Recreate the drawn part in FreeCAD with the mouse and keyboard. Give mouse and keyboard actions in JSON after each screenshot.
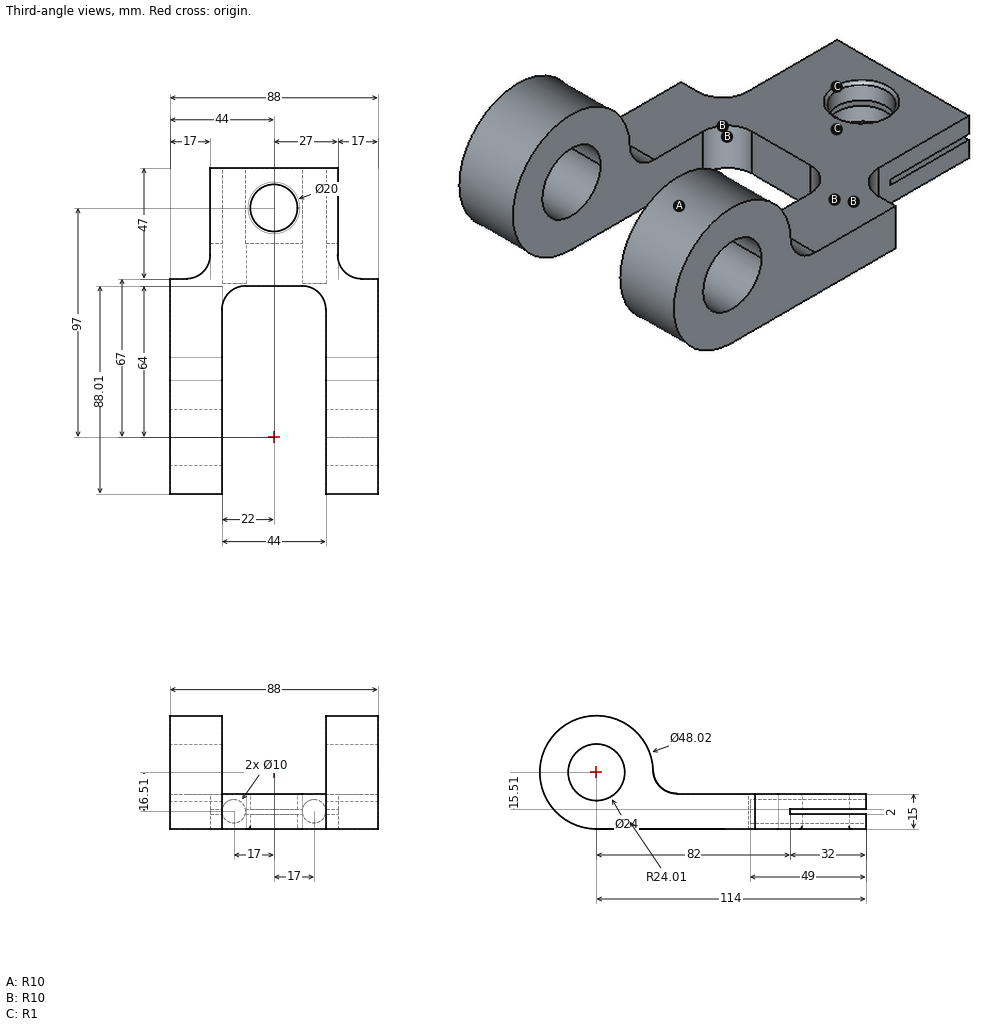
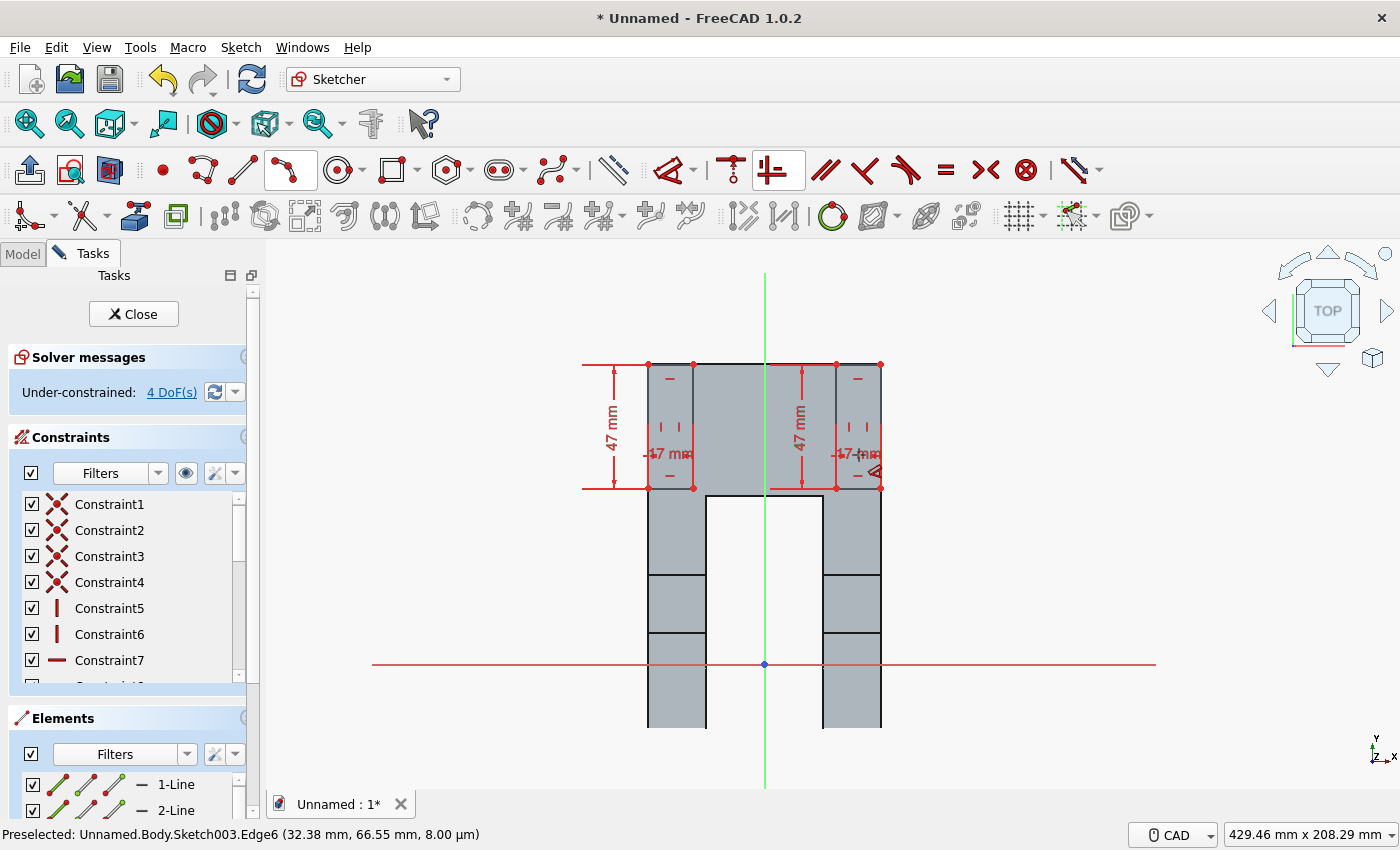
{"action": "left_click", "coordinate": [648, 365]}
{"action": "left_click", "coordinate": [706, 699]}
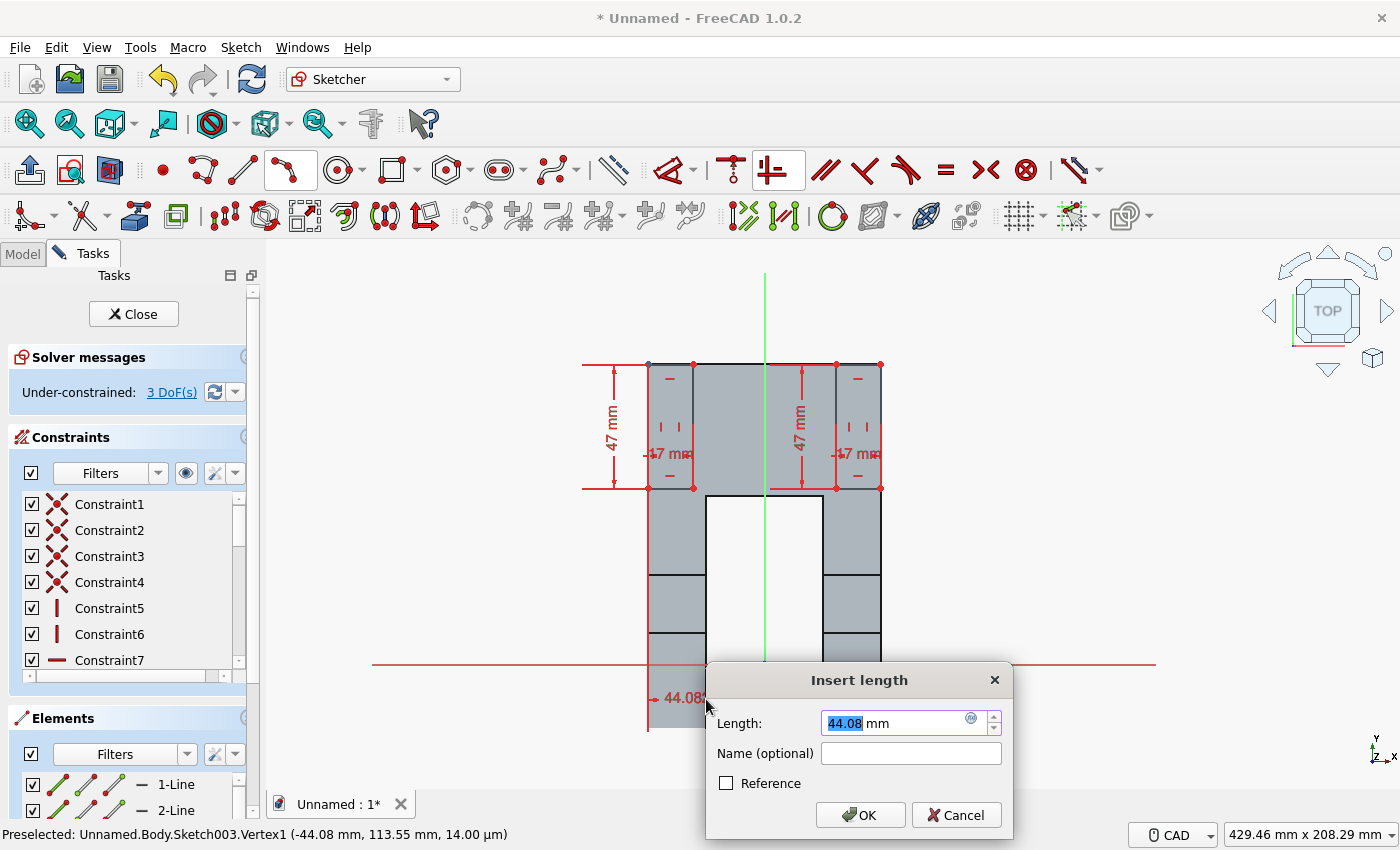
{"action": "type", "text": "44"}
{"action": "key", "text": "Return"}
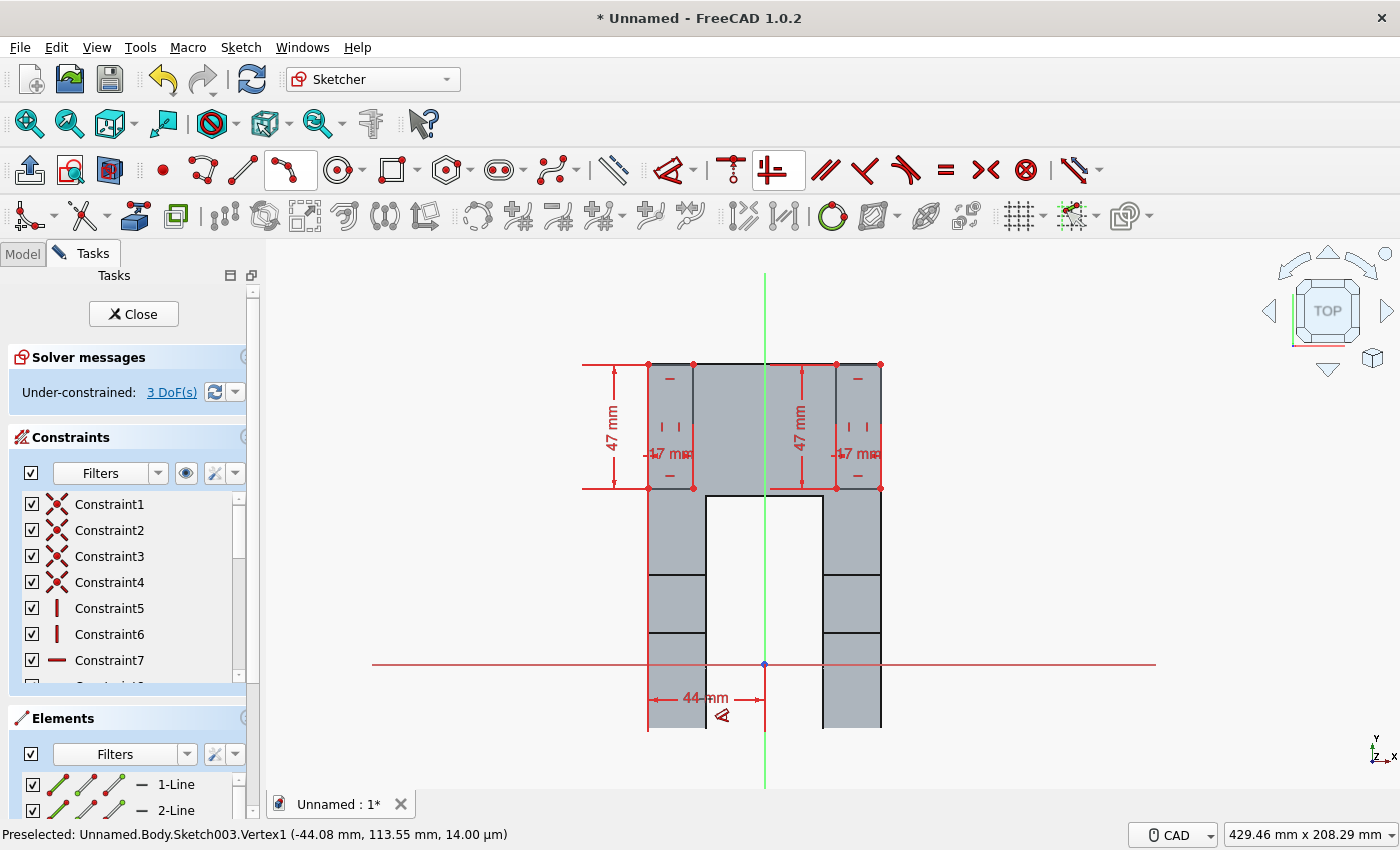
{"action": "left_click", "coordinate": [648, 489]}
{"action": "left_click", "coordinate": [614, 577]}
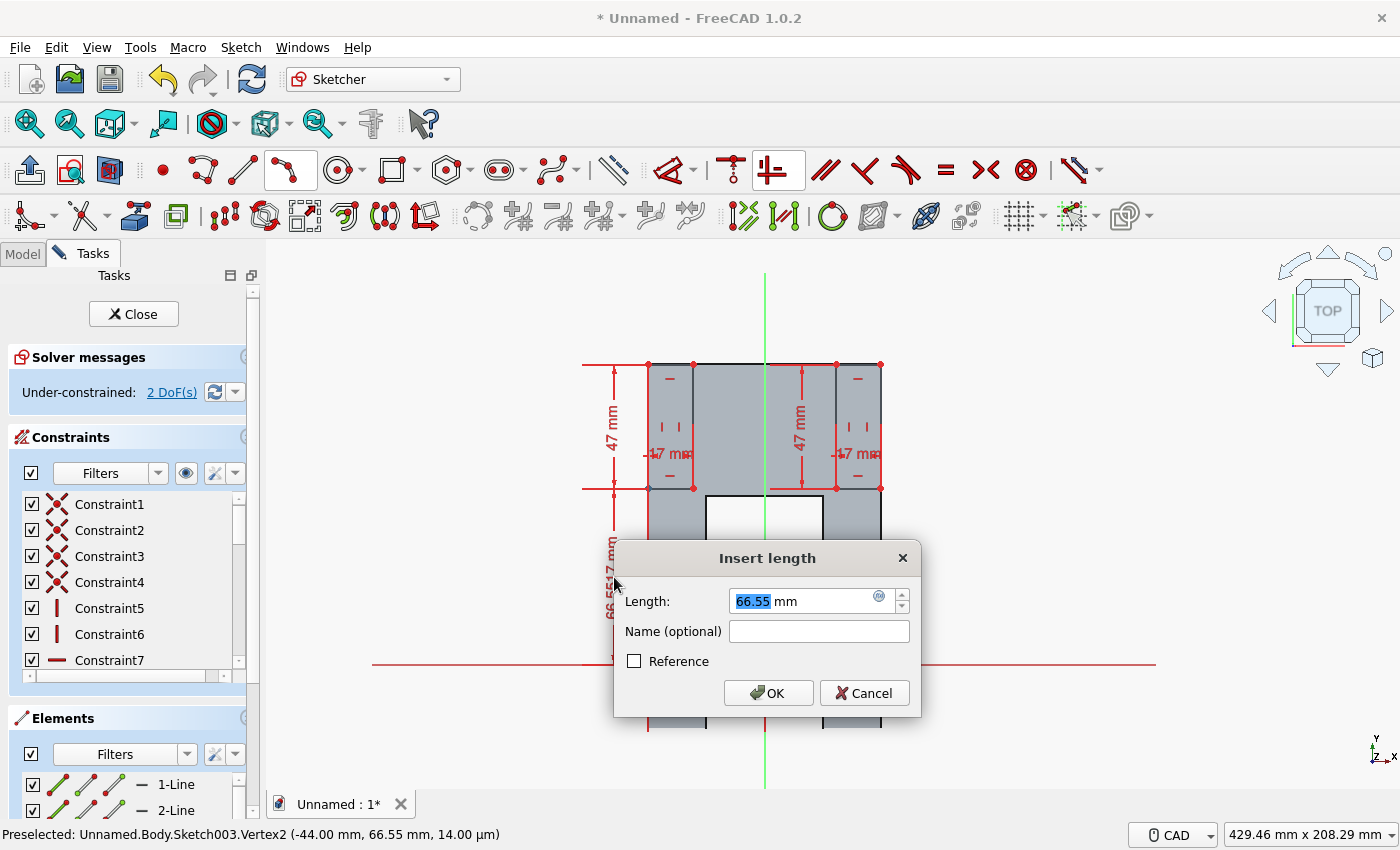
{"action": "type", "text": "67"}
{"action": "key", "text": "Return"}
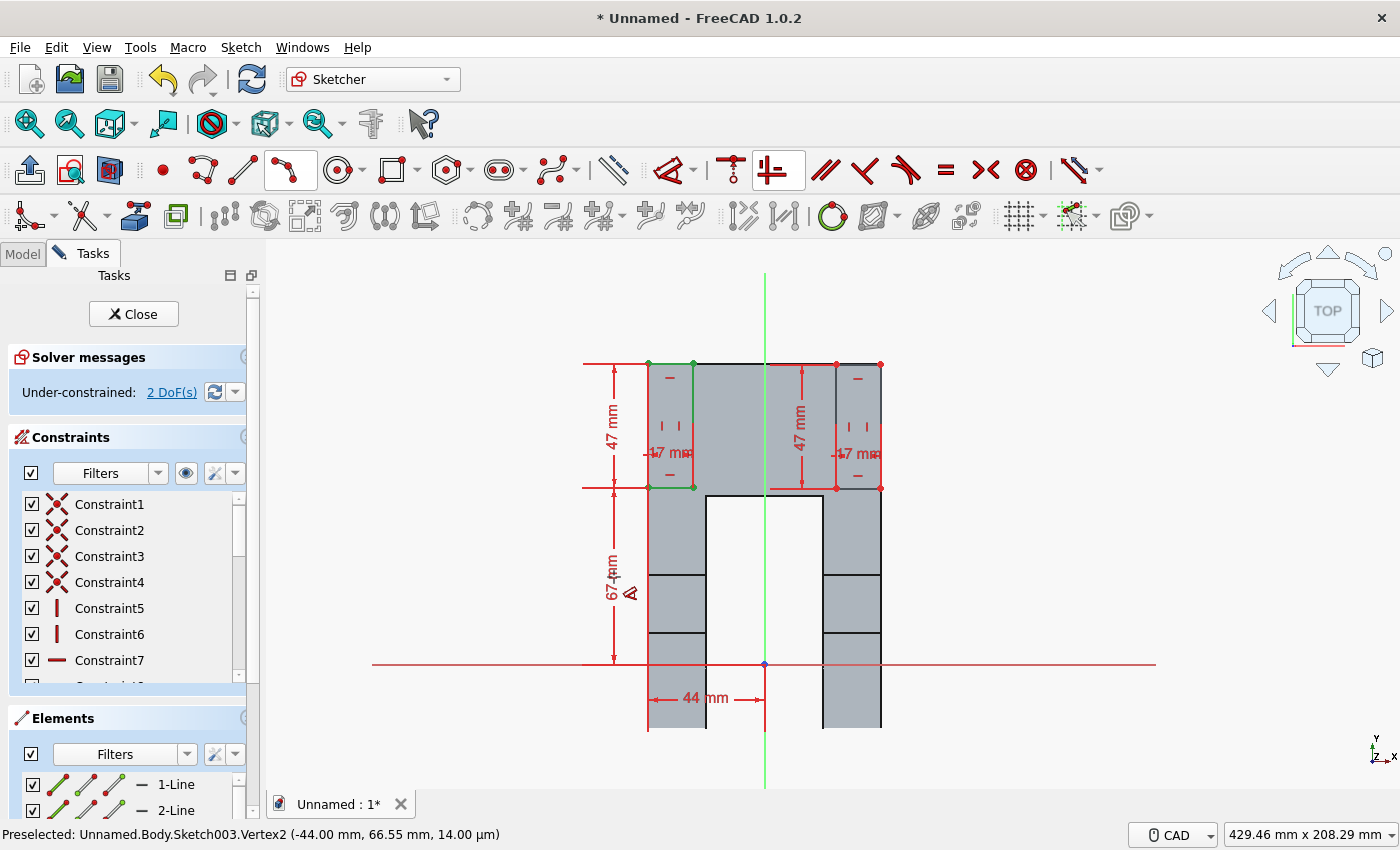
{"action": "left_click", "coordinate": [836, 365]}
{"action": "left_click", "coordinate": [800, 699]}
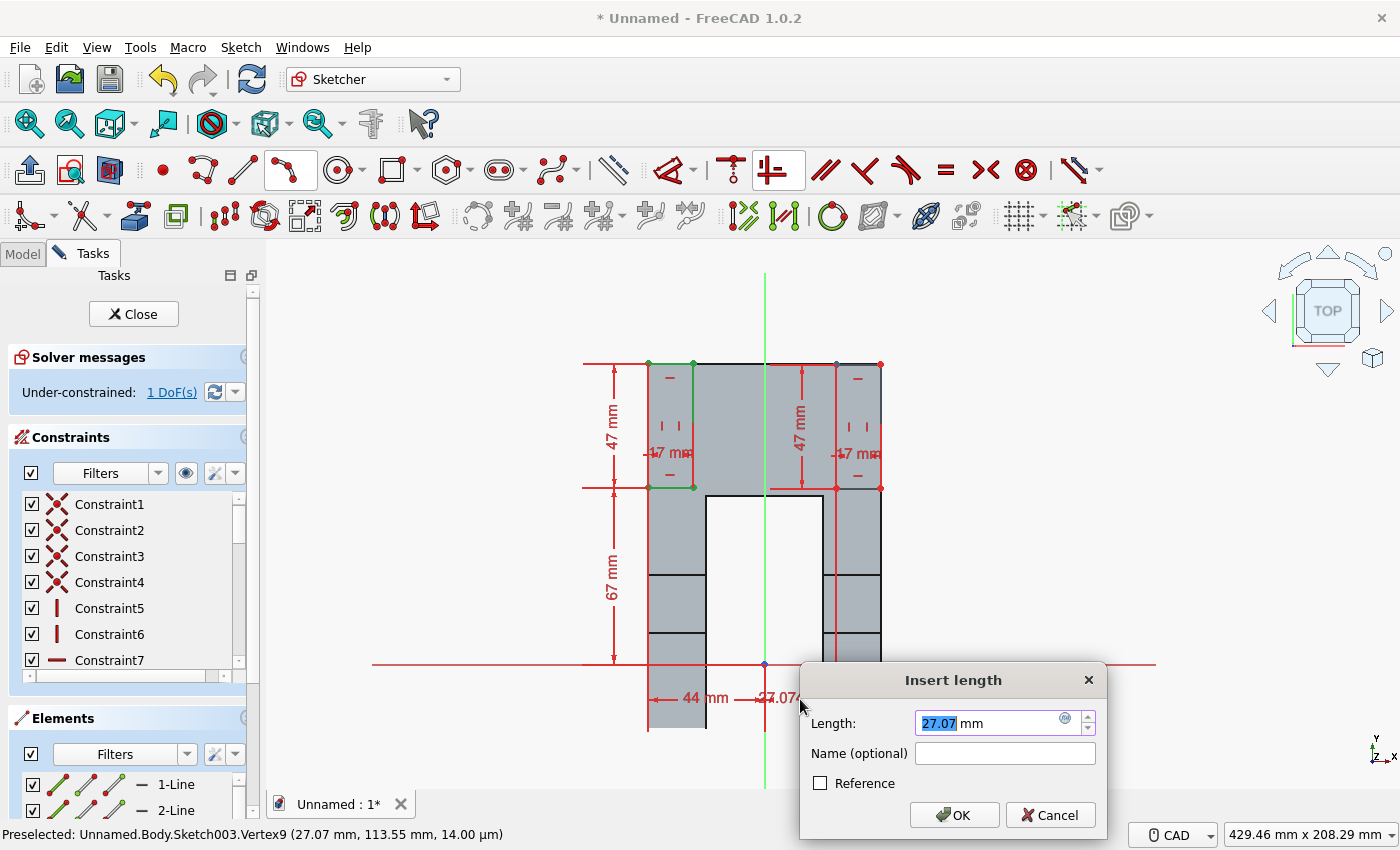
{"action": "type", "text": "27"}
{"action": "key", "text": "Return"}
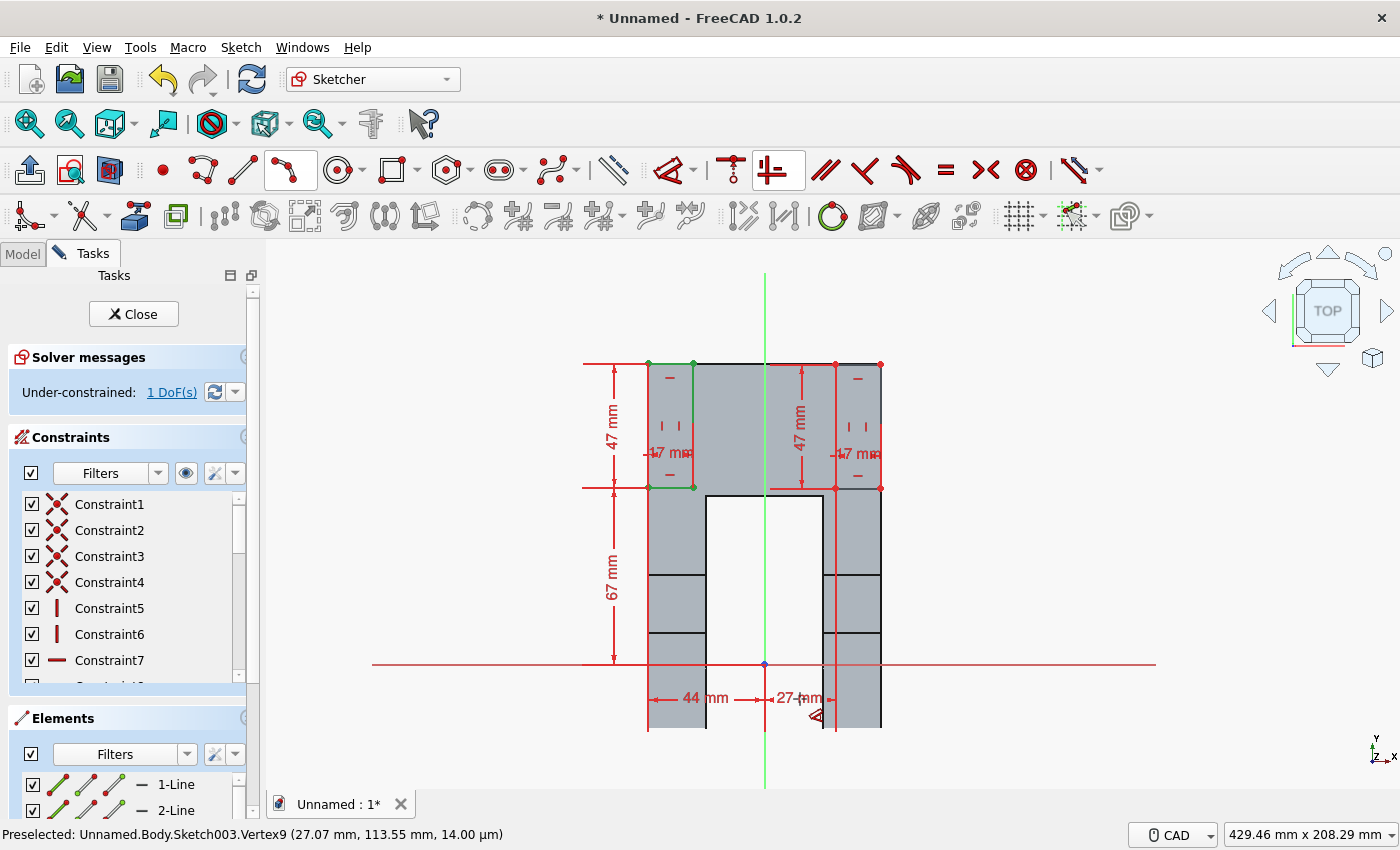
{"action": "left_click", "coordinate": [836, 489]}
{"action": "left_click", "coordinate": [870, 577]}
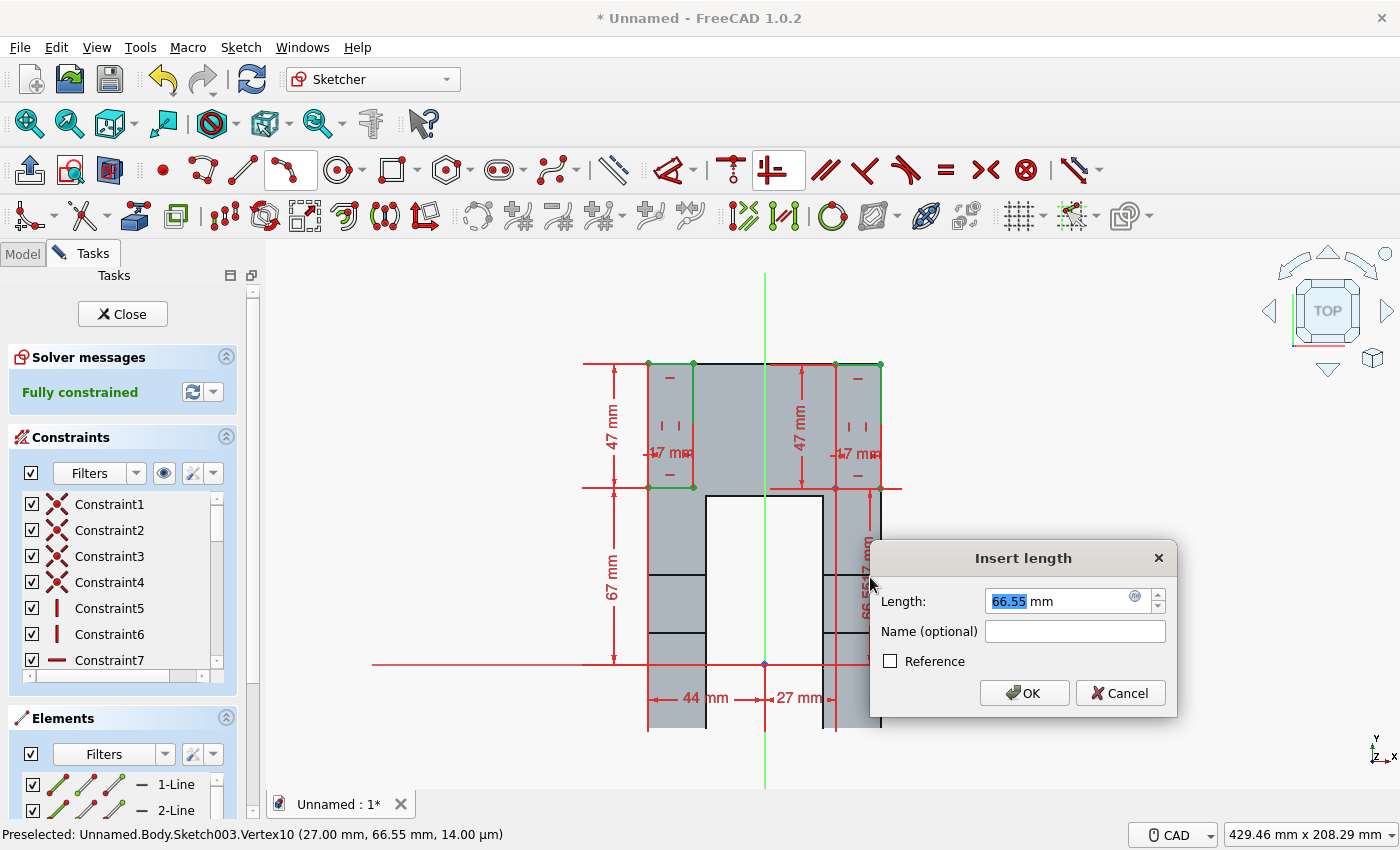
{"action": "type", "text": "67"}
{"action": "key", "text": "Return"}
{"action": "key", "text": "Escape"}